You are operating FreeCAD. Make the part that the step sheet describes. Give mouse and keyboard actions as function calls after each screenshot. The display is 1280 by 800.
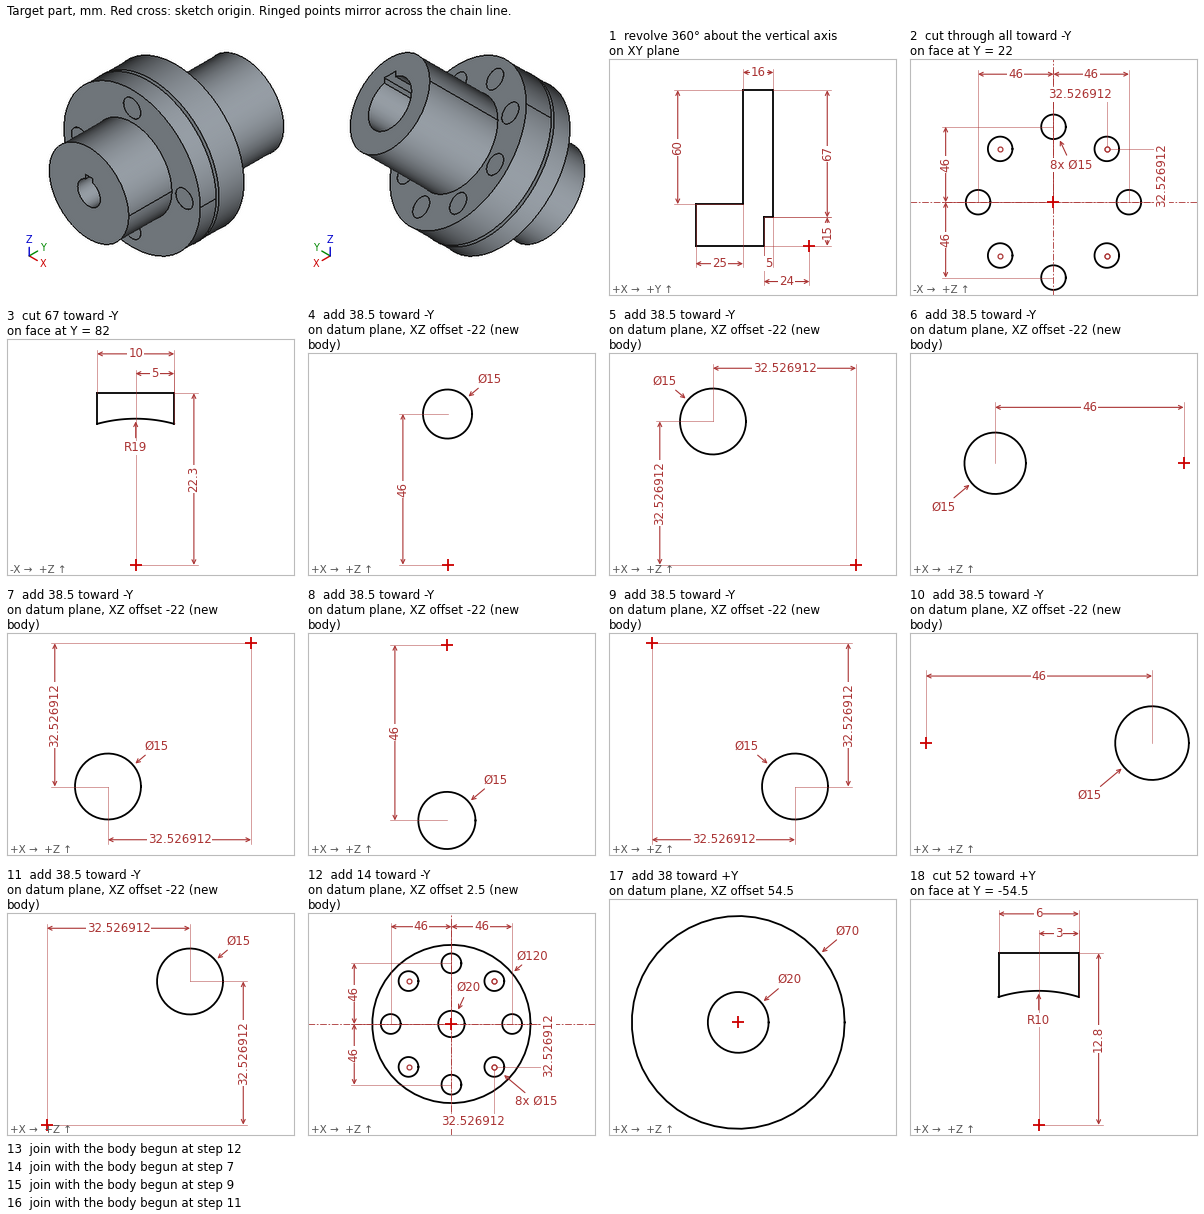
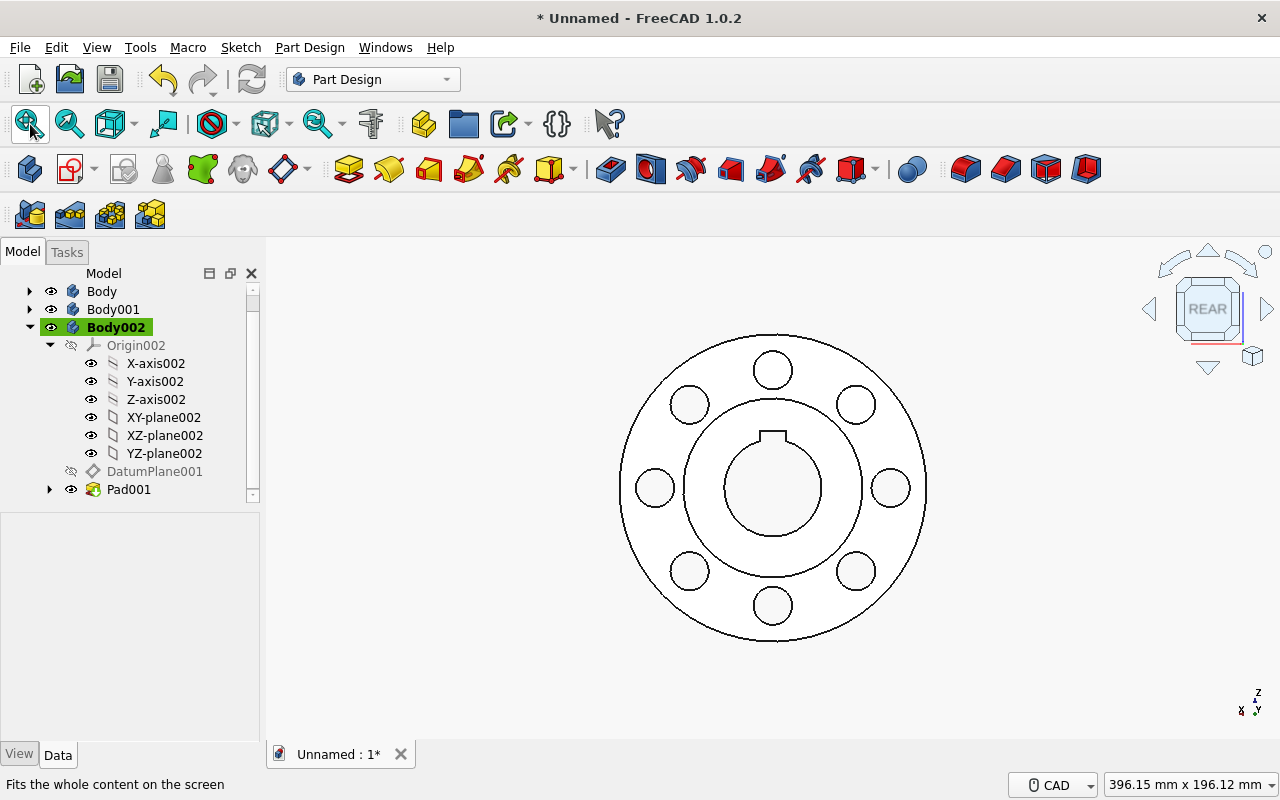
click(30, 170)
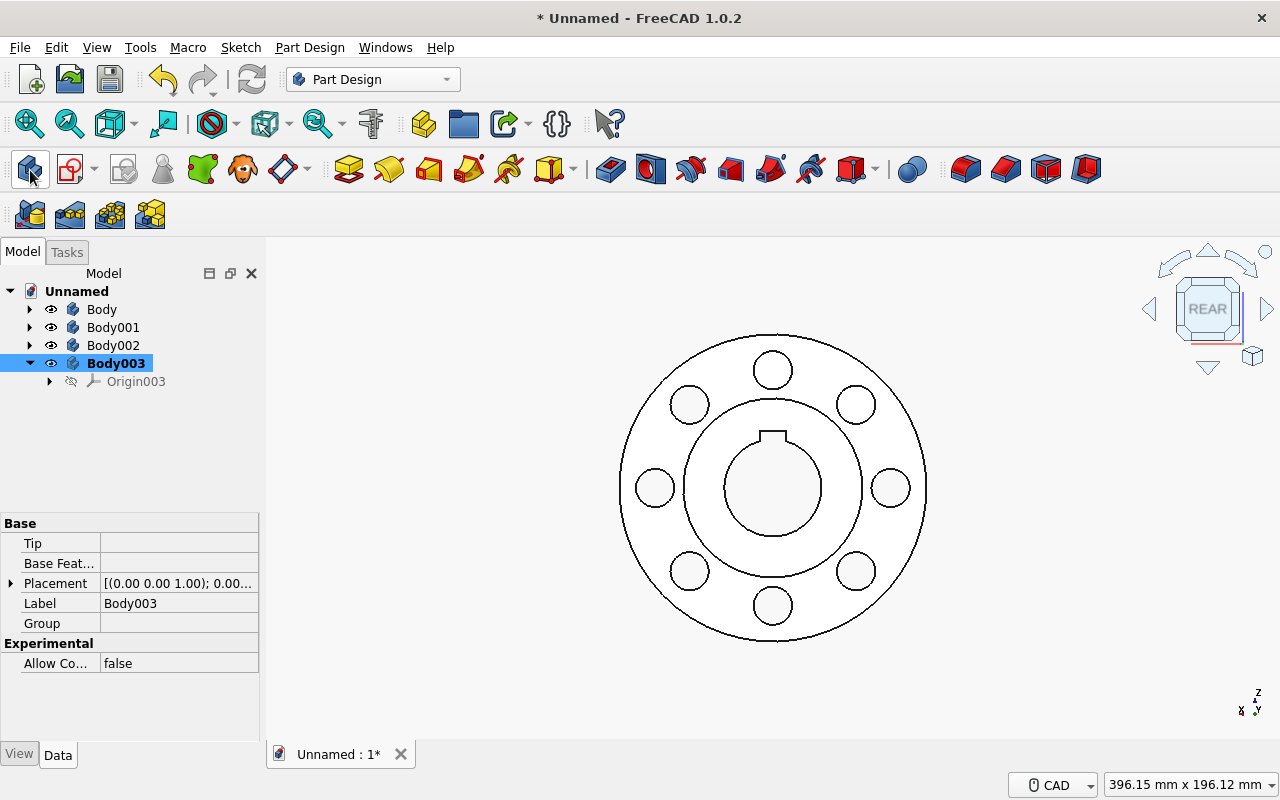
click(50, 381)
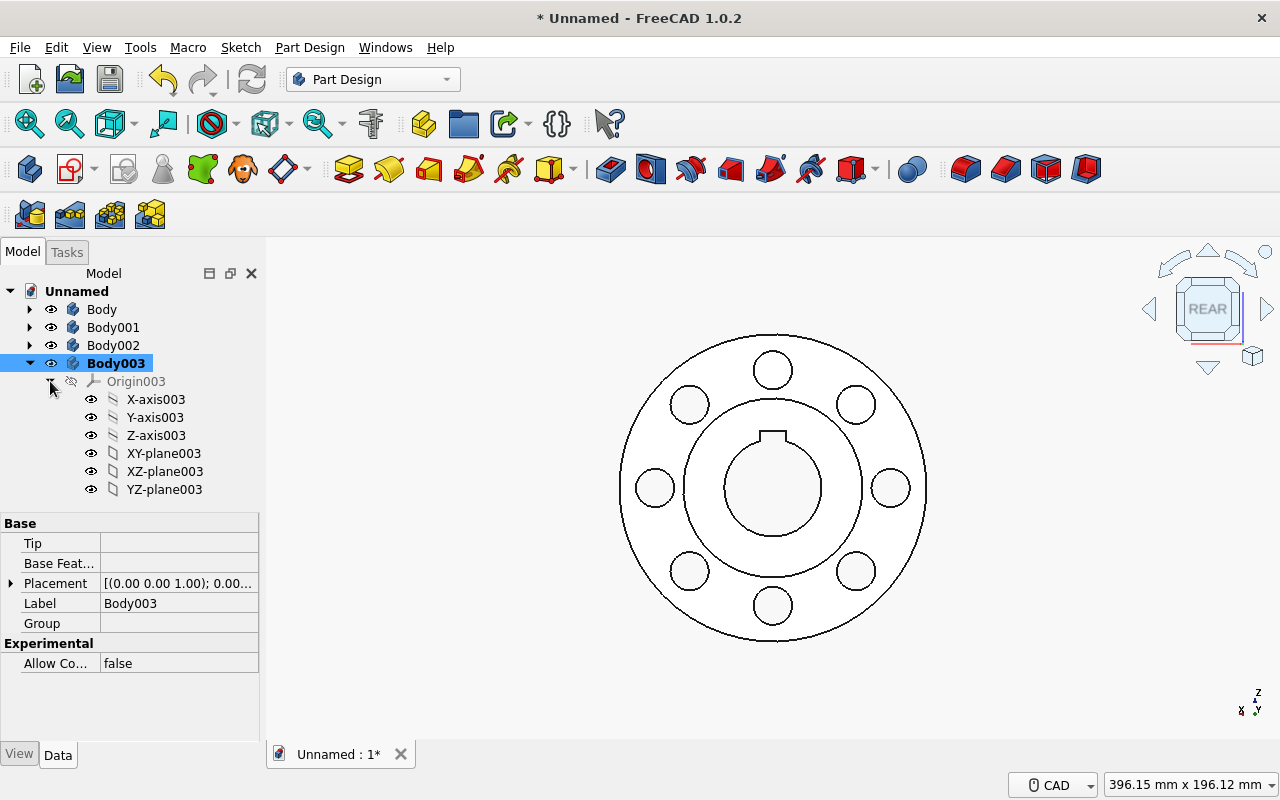
click(136, 471)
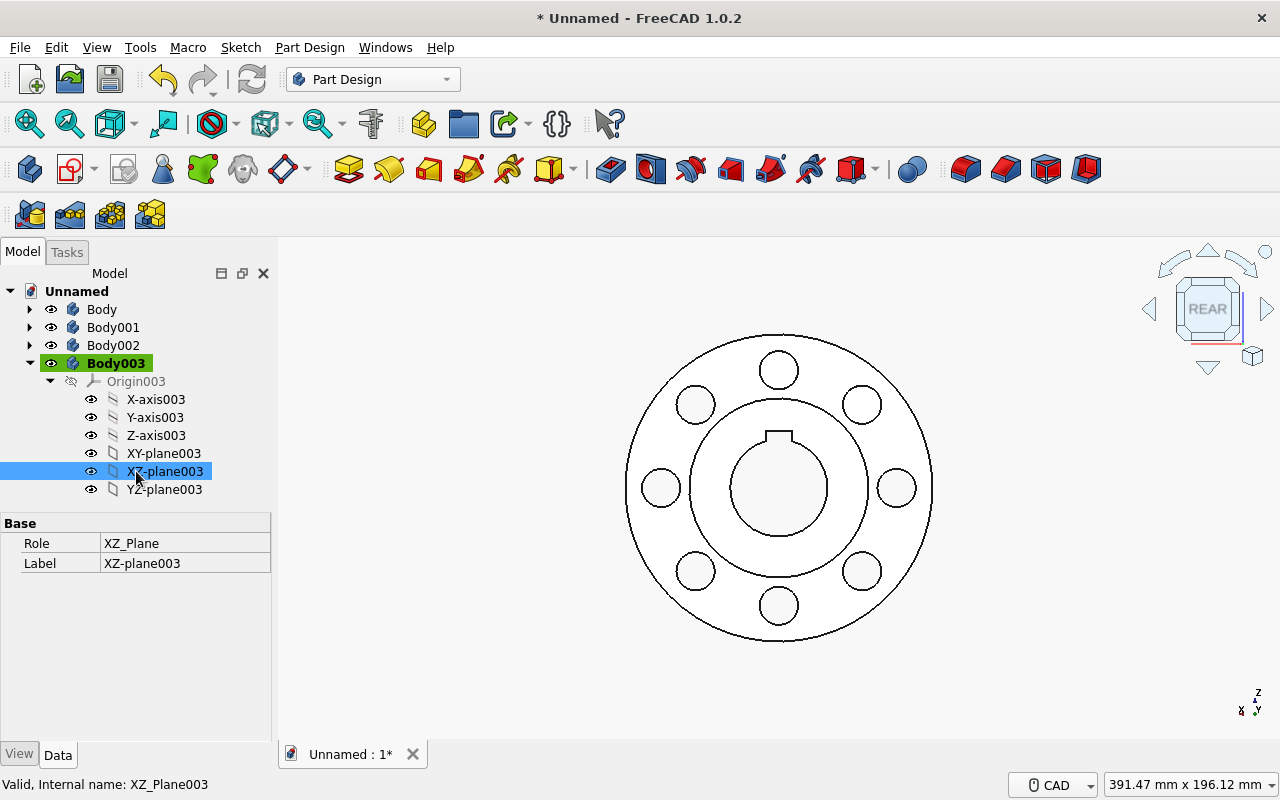
click(284, 170)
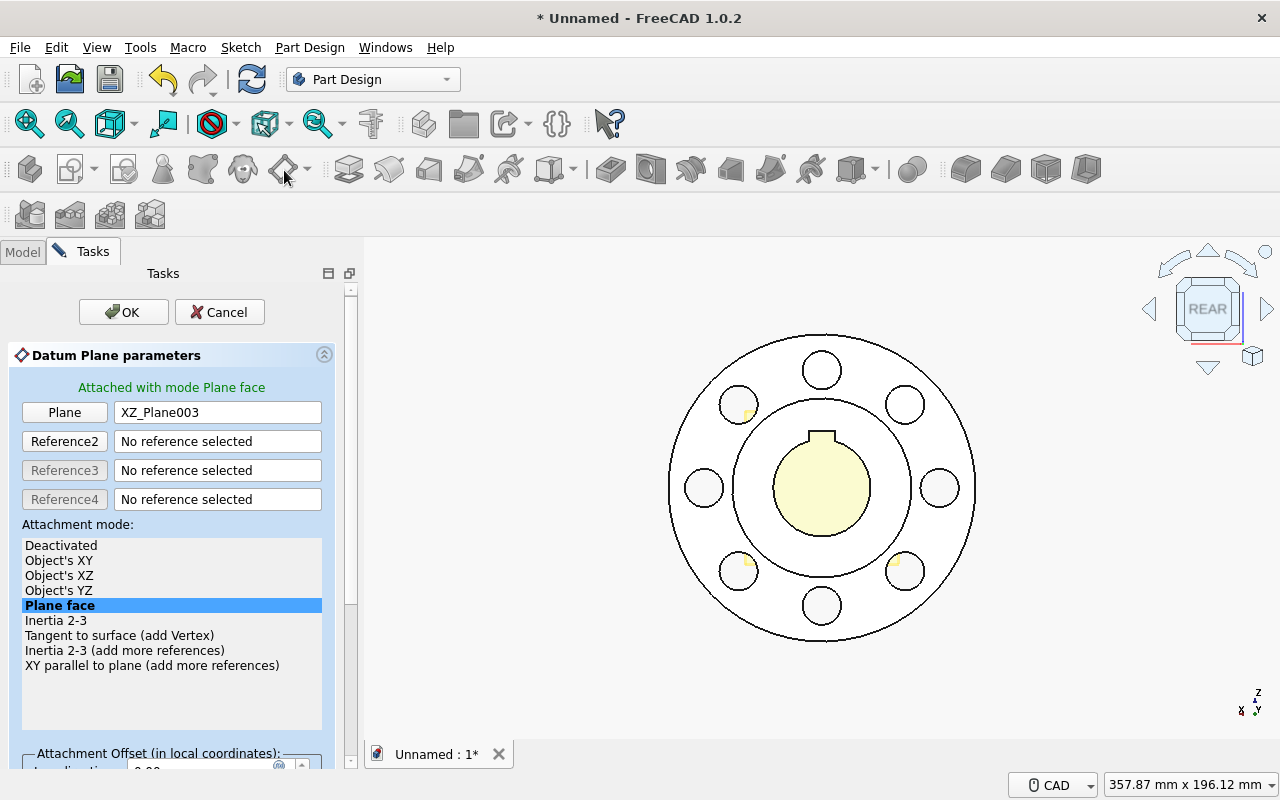
scroll(351, 526, down, 3)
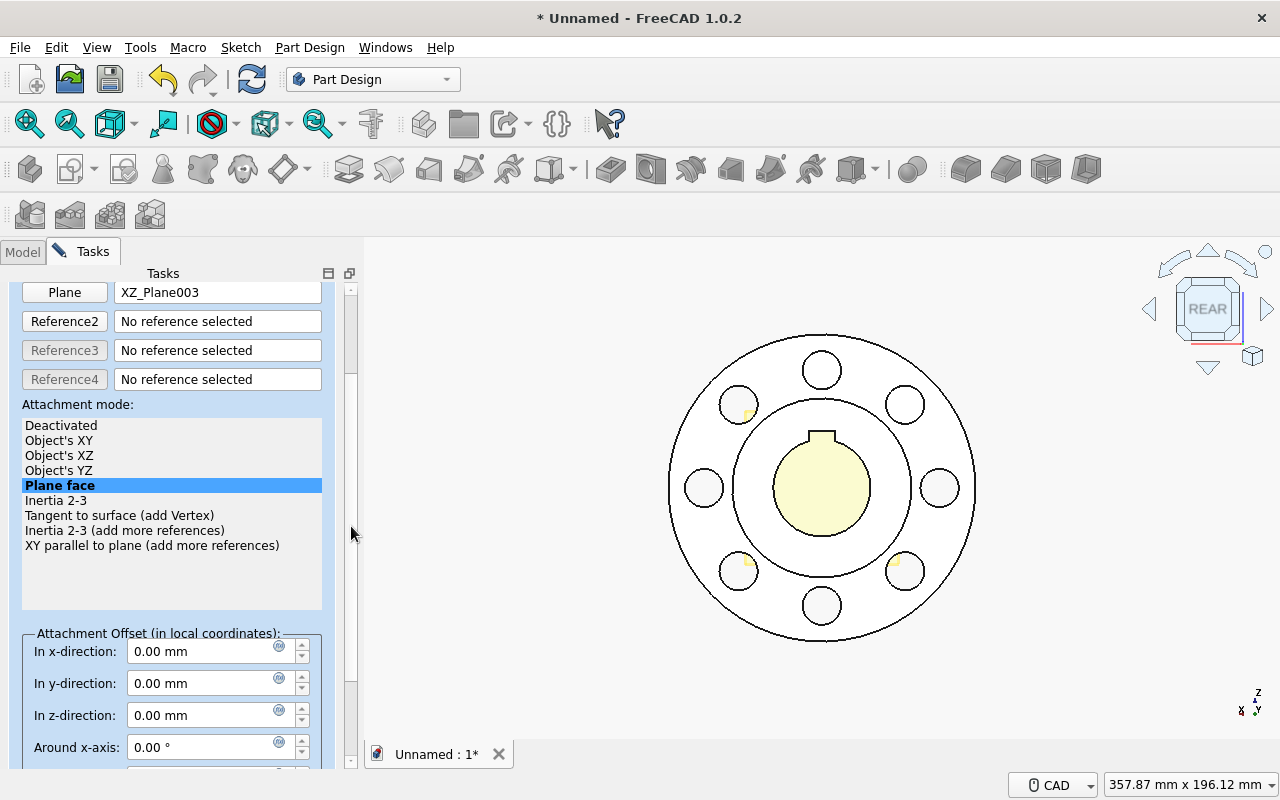
triple_click(210, 655)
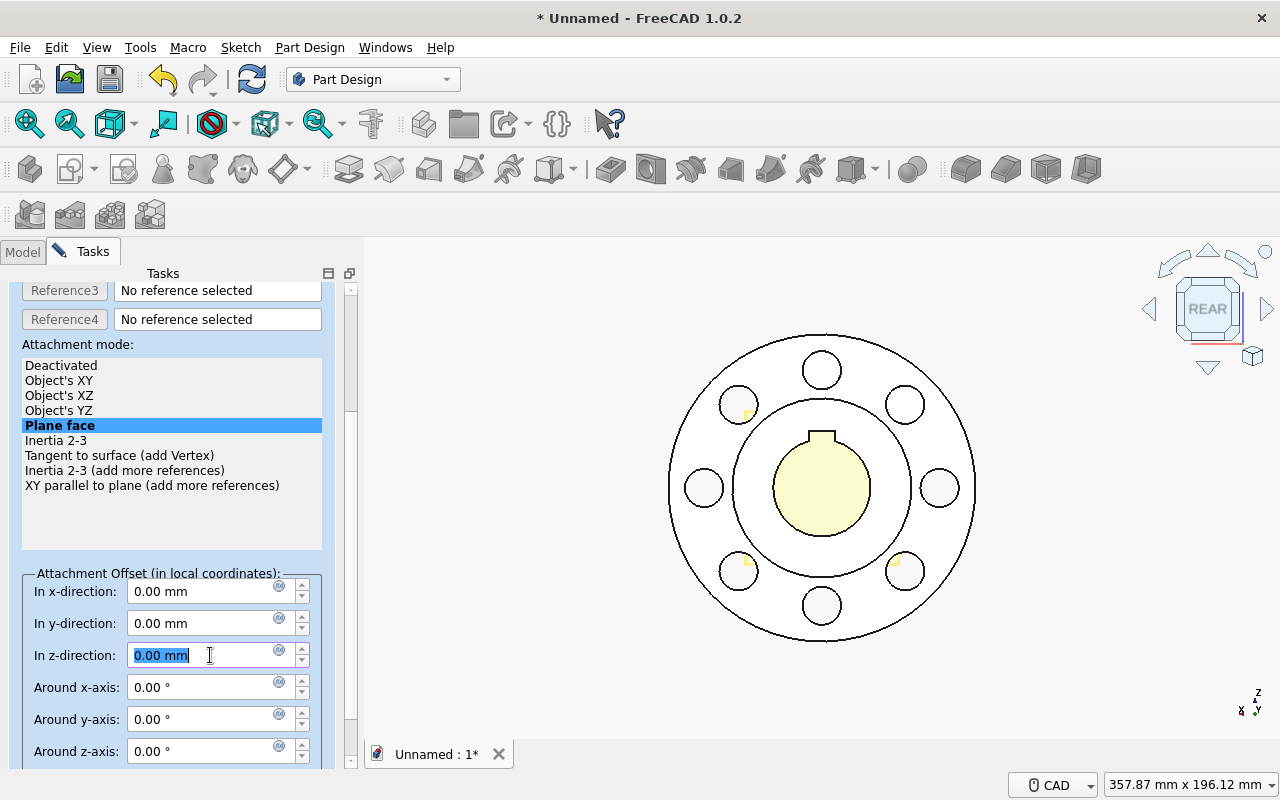
text(-22)
key(Tab)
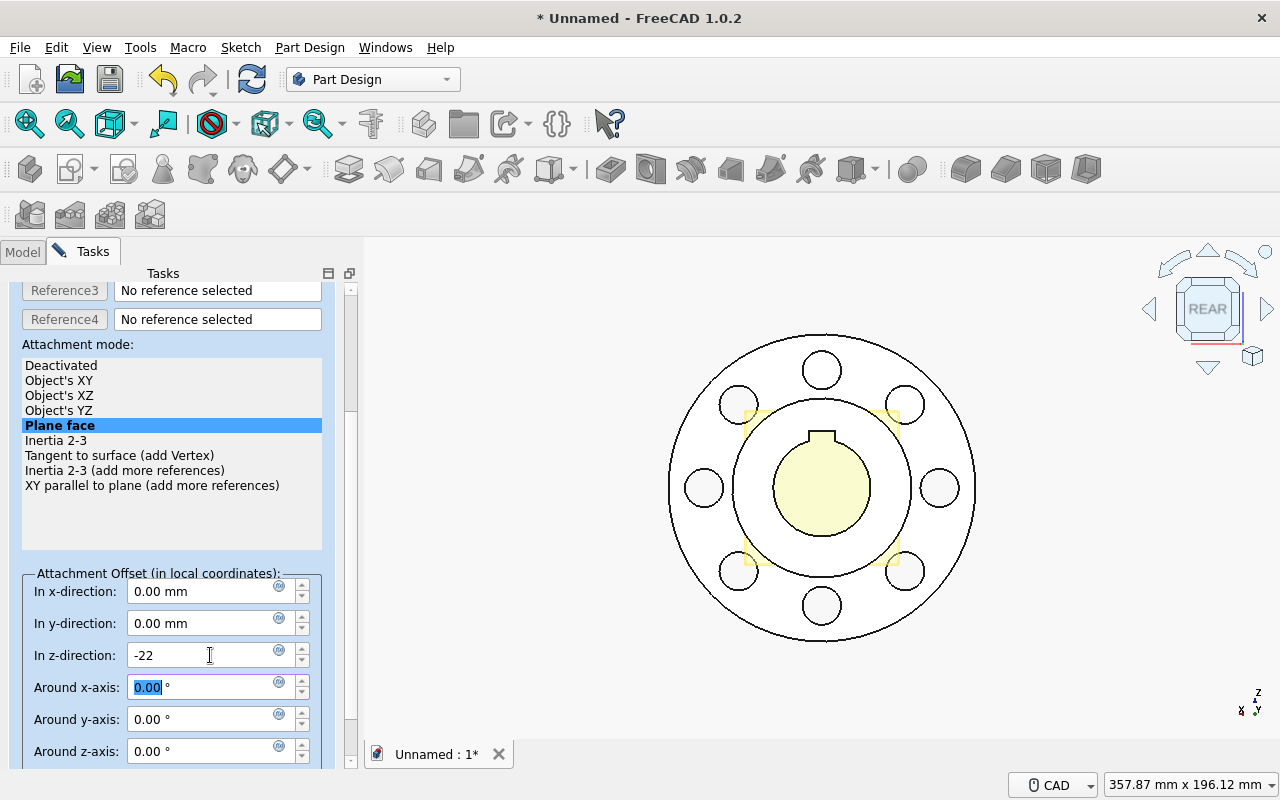
scroll(351, 526, up, 4)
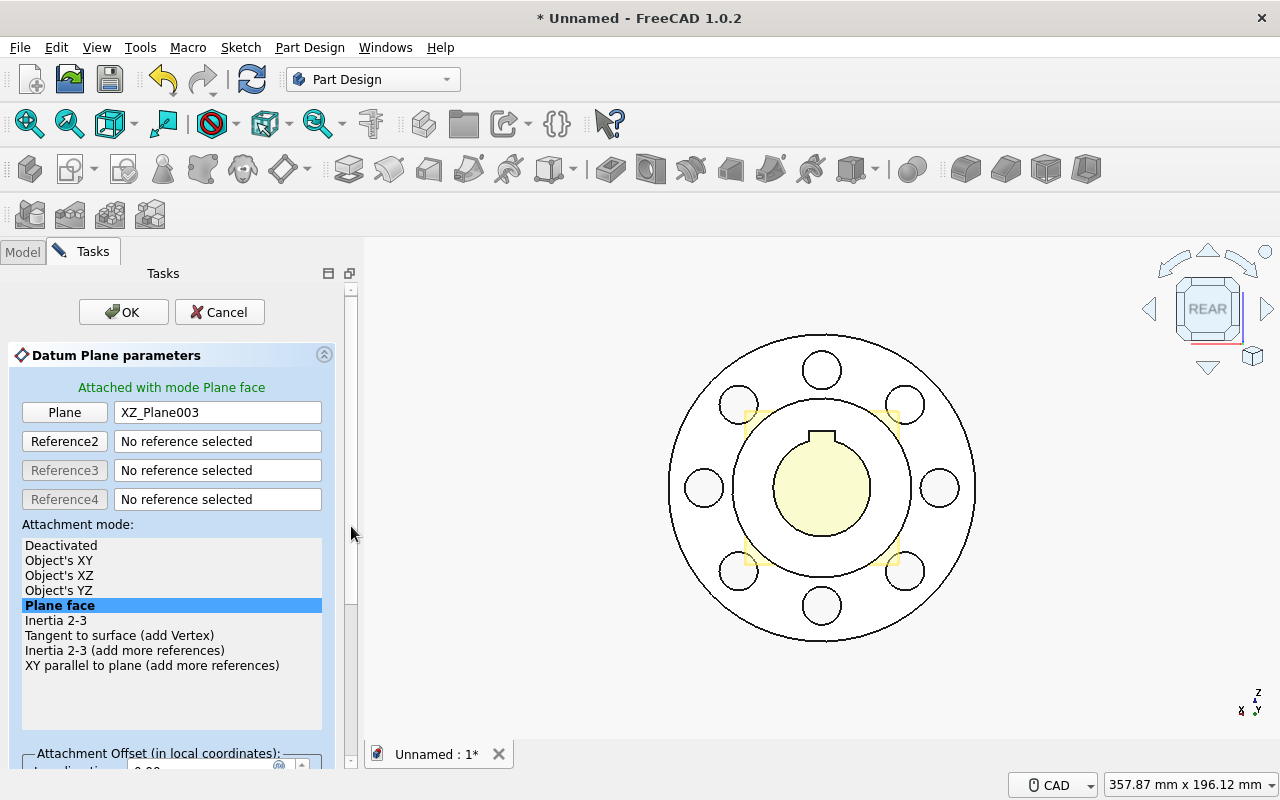
click(124, 312)